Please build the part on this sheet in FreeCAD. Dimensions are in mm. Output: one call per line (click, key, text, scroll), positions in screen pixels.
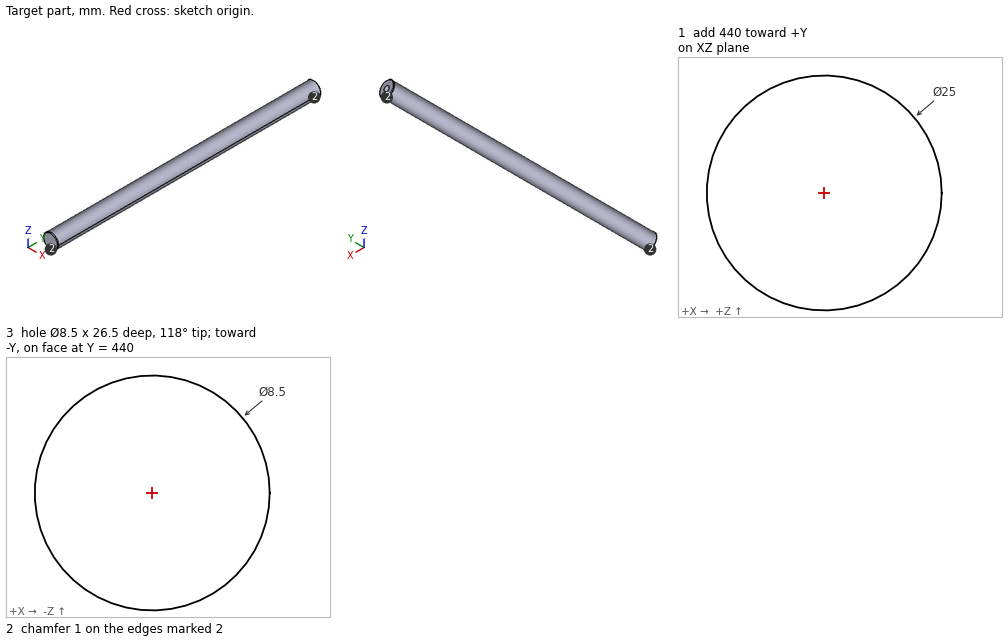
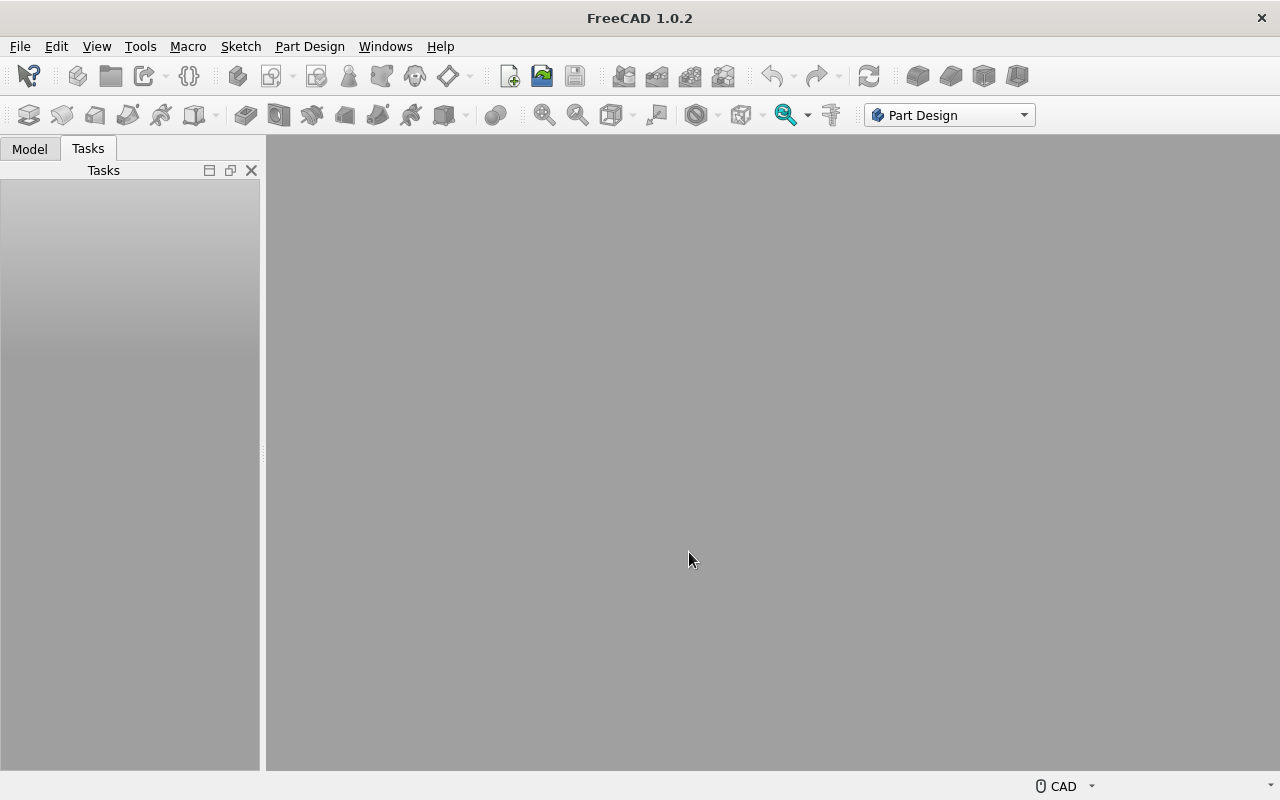
click(509, 76)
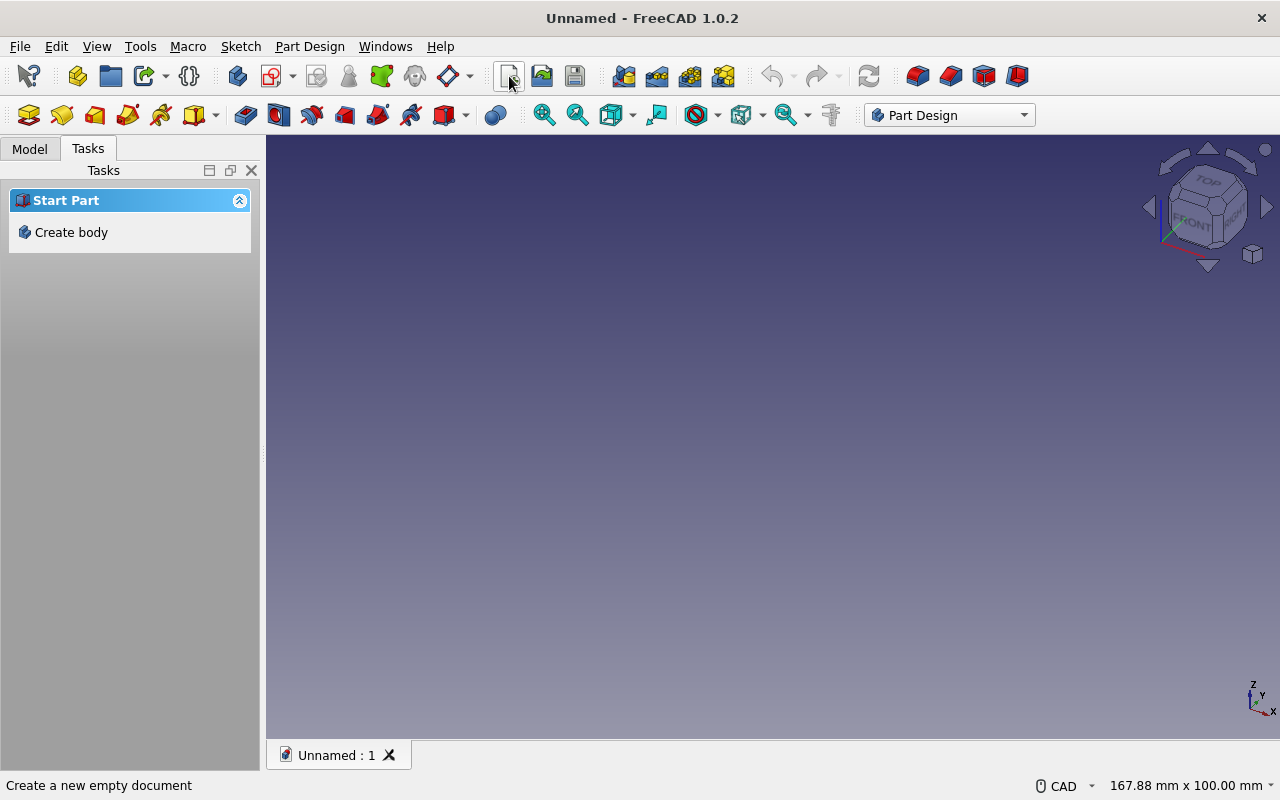
click(270, 76)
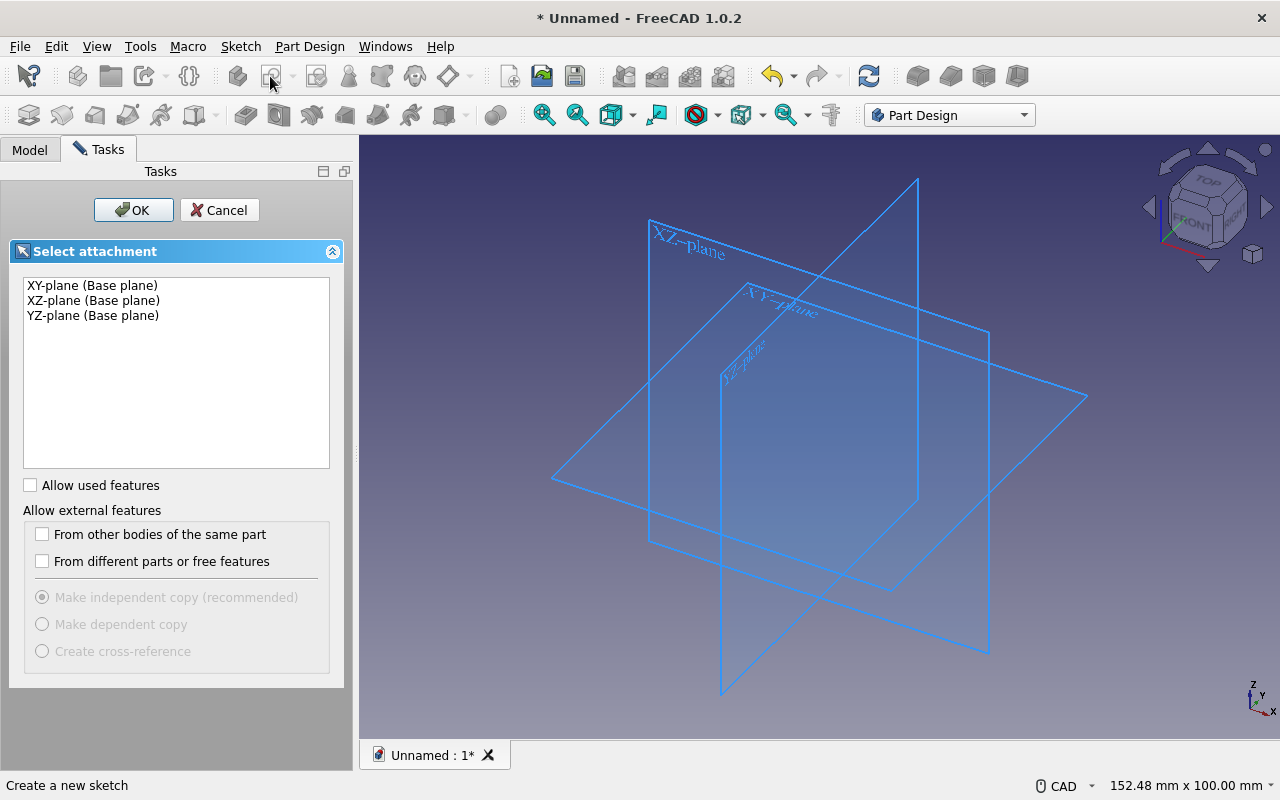
click(84, 300)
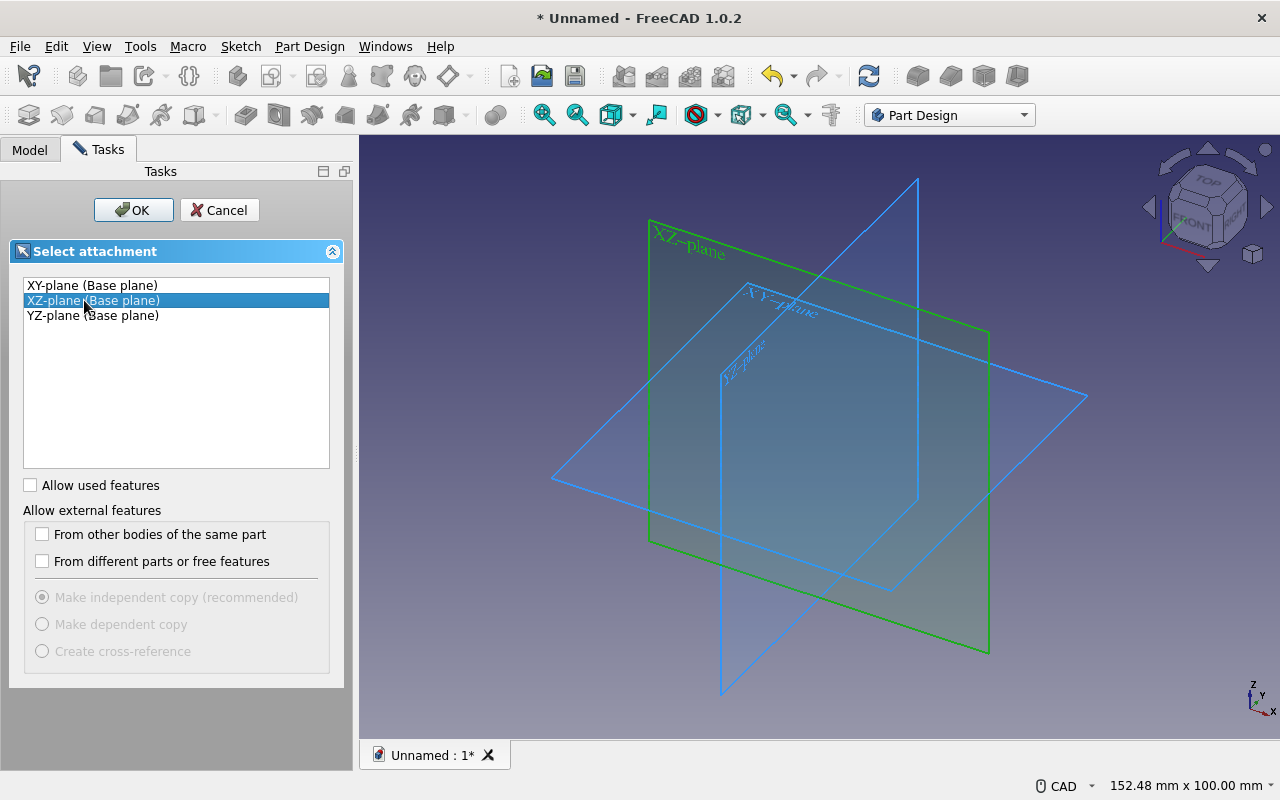
click(134, 210)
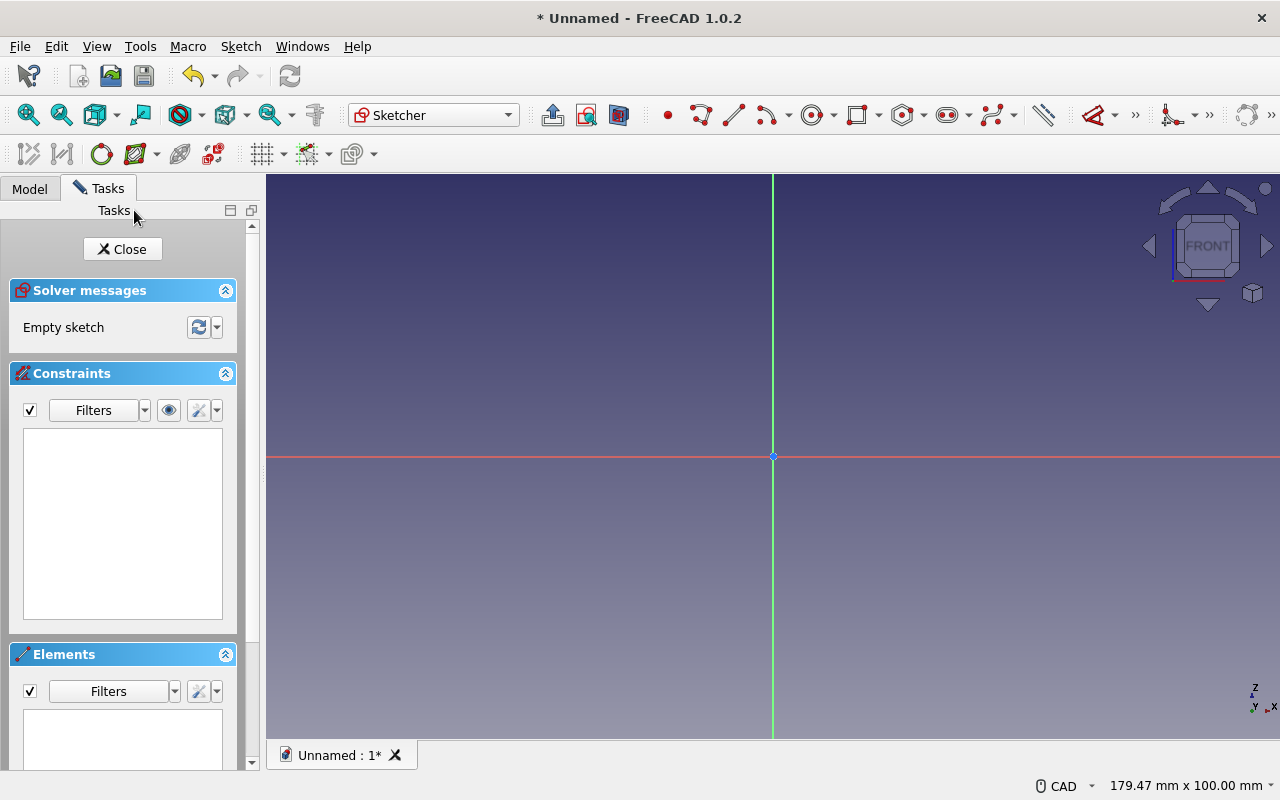
scroll(813, 456, up, 5)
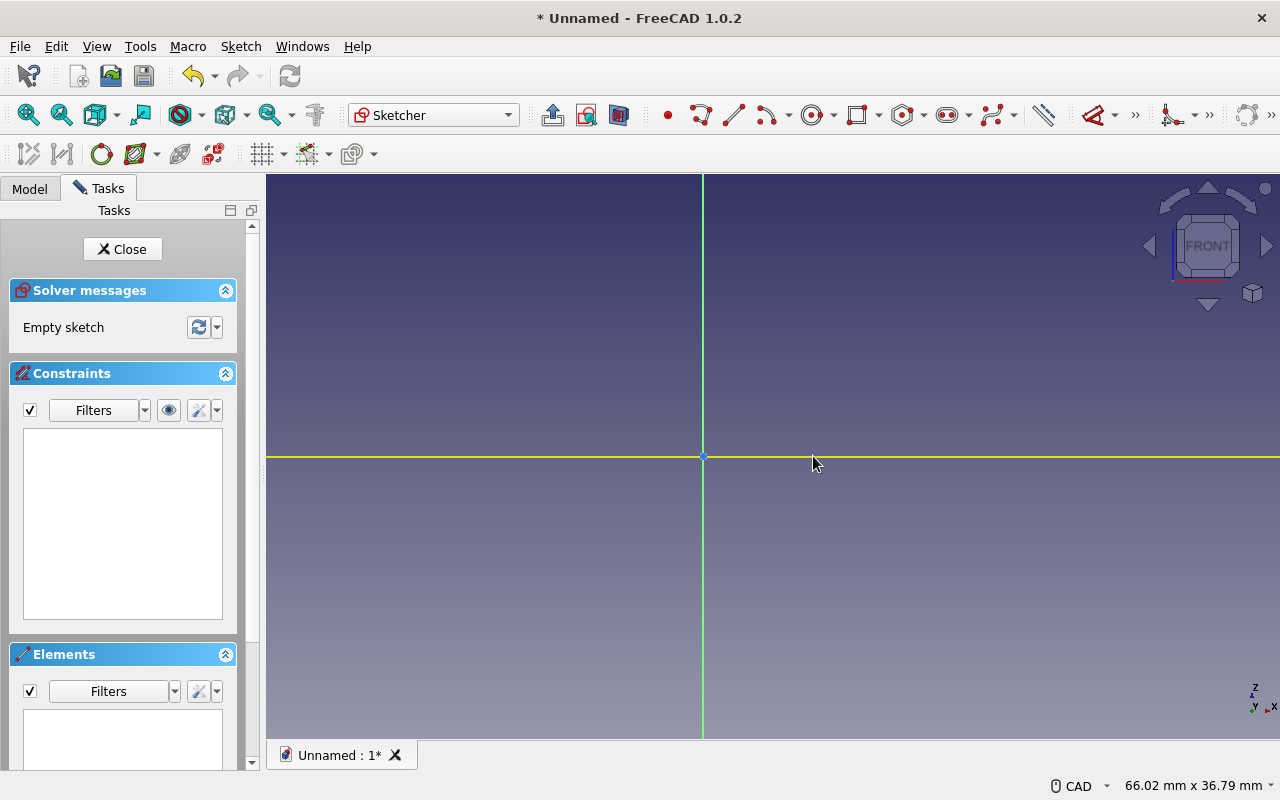
key(g)
key(c)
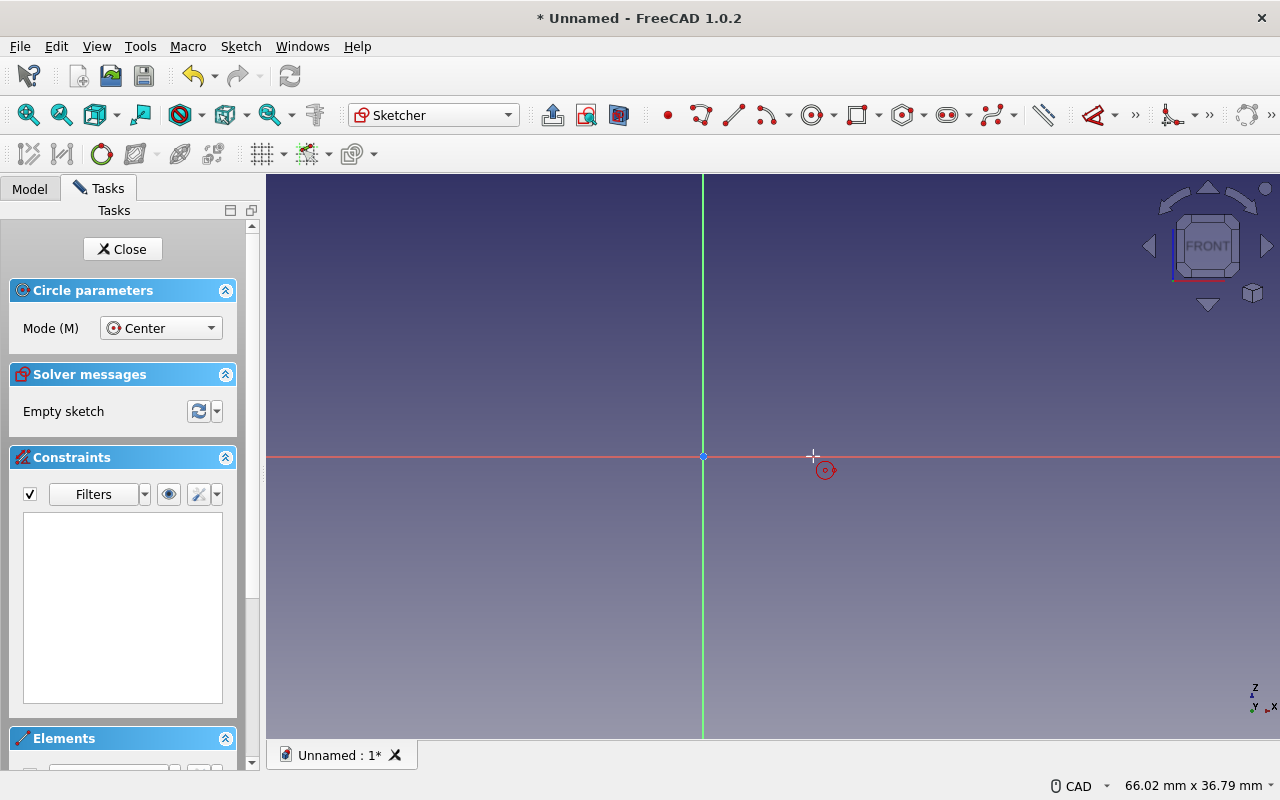
click(703, 456)
move(839, 321)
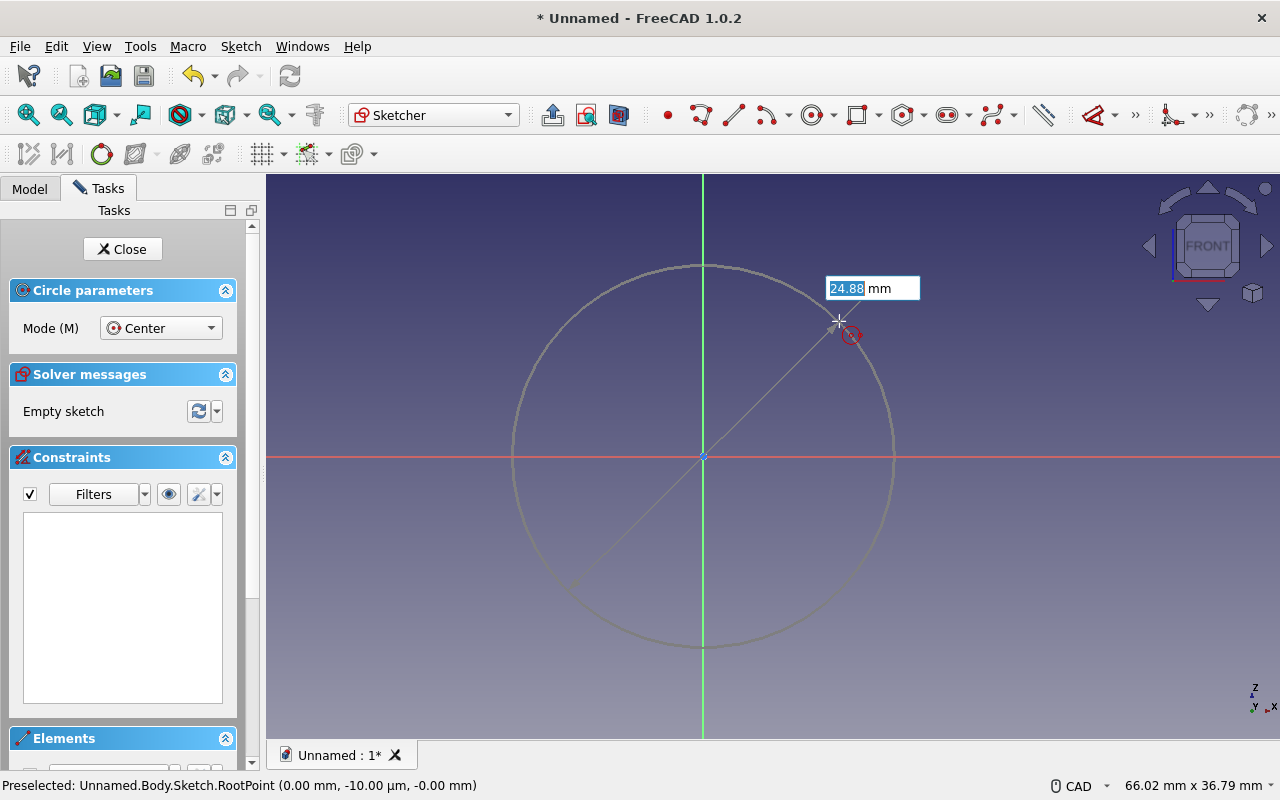
text(25)
key(Return)
key(Escape)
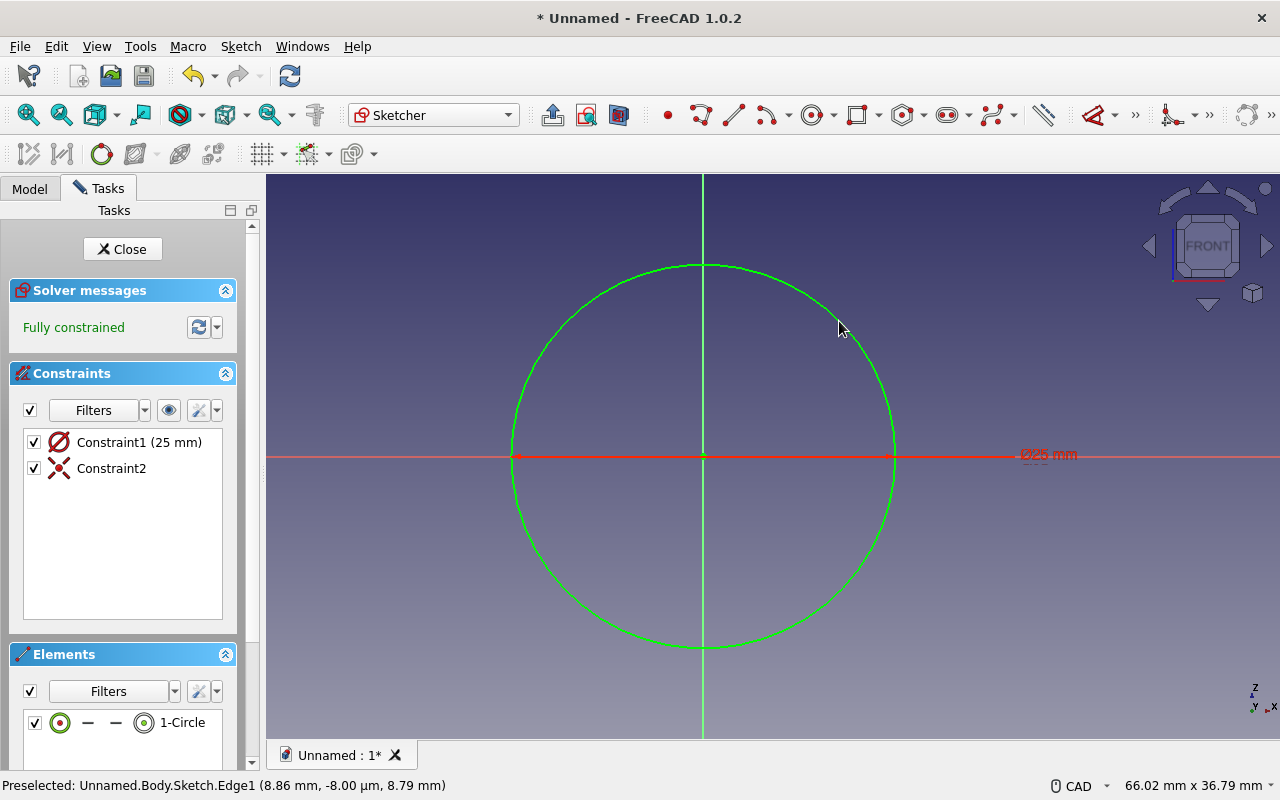
click(123, 249)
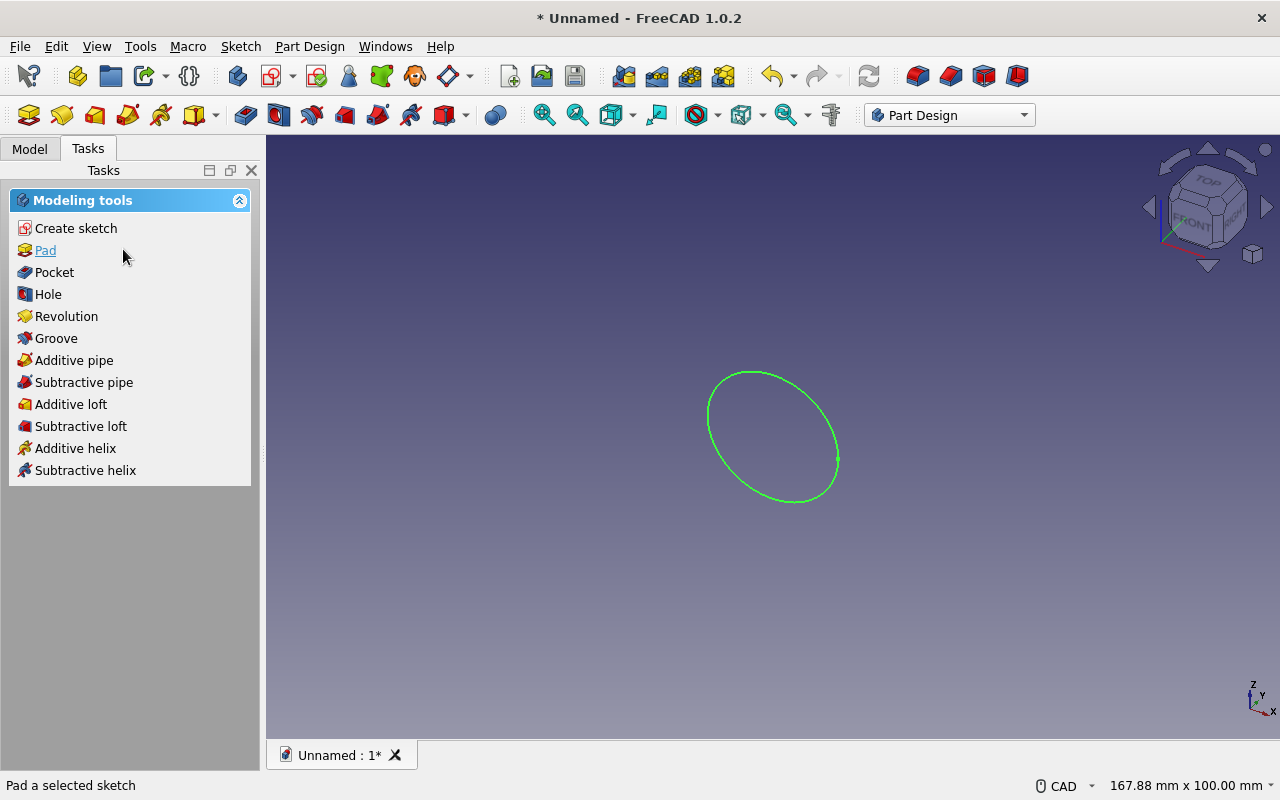
click(29, 116)